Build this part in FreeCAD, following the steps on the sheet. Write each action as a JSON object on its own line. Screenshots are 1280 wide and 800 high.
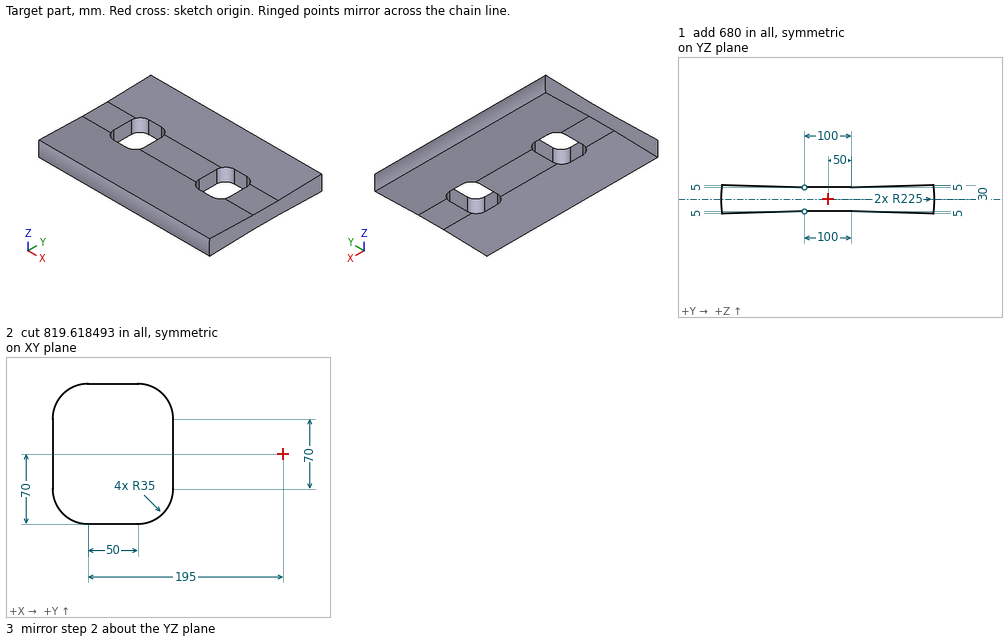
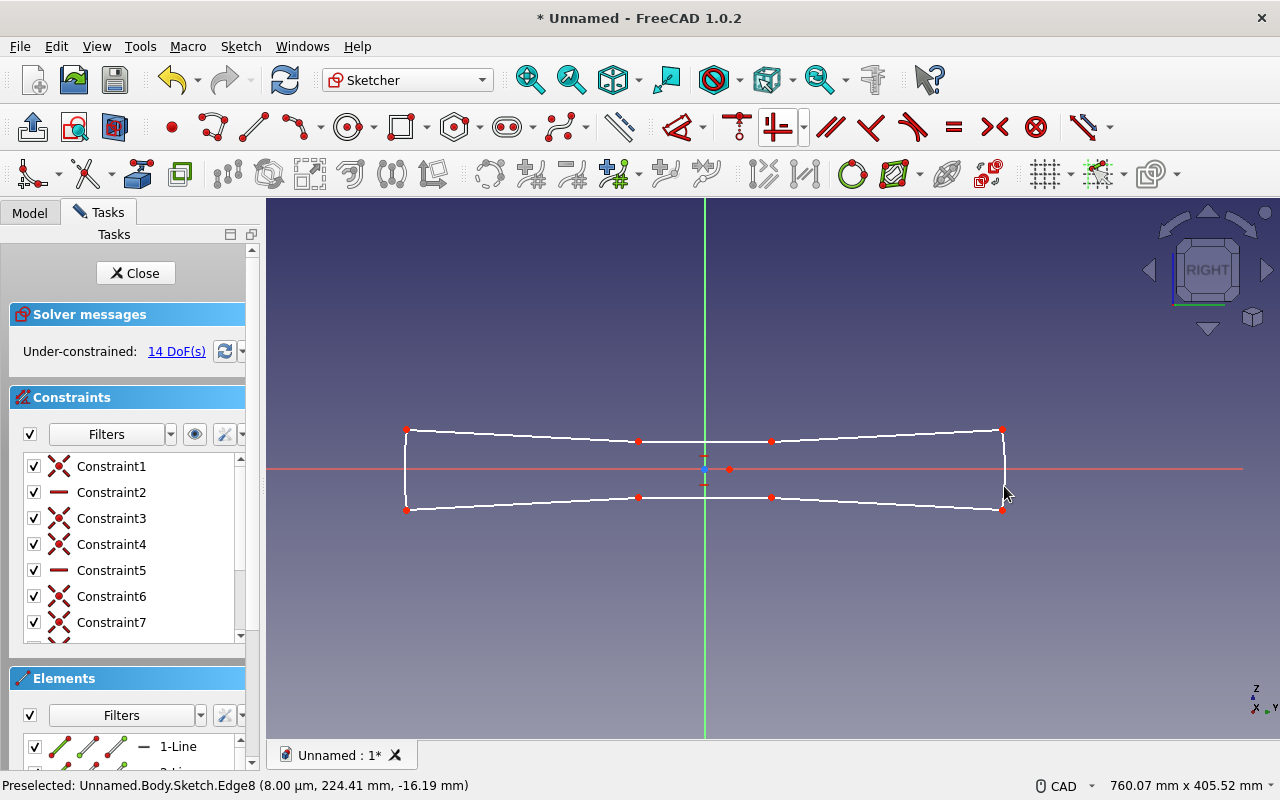
{"action": "left_click_drag", "start_coordinate": [695, 459], "coordinate": [739, 480]}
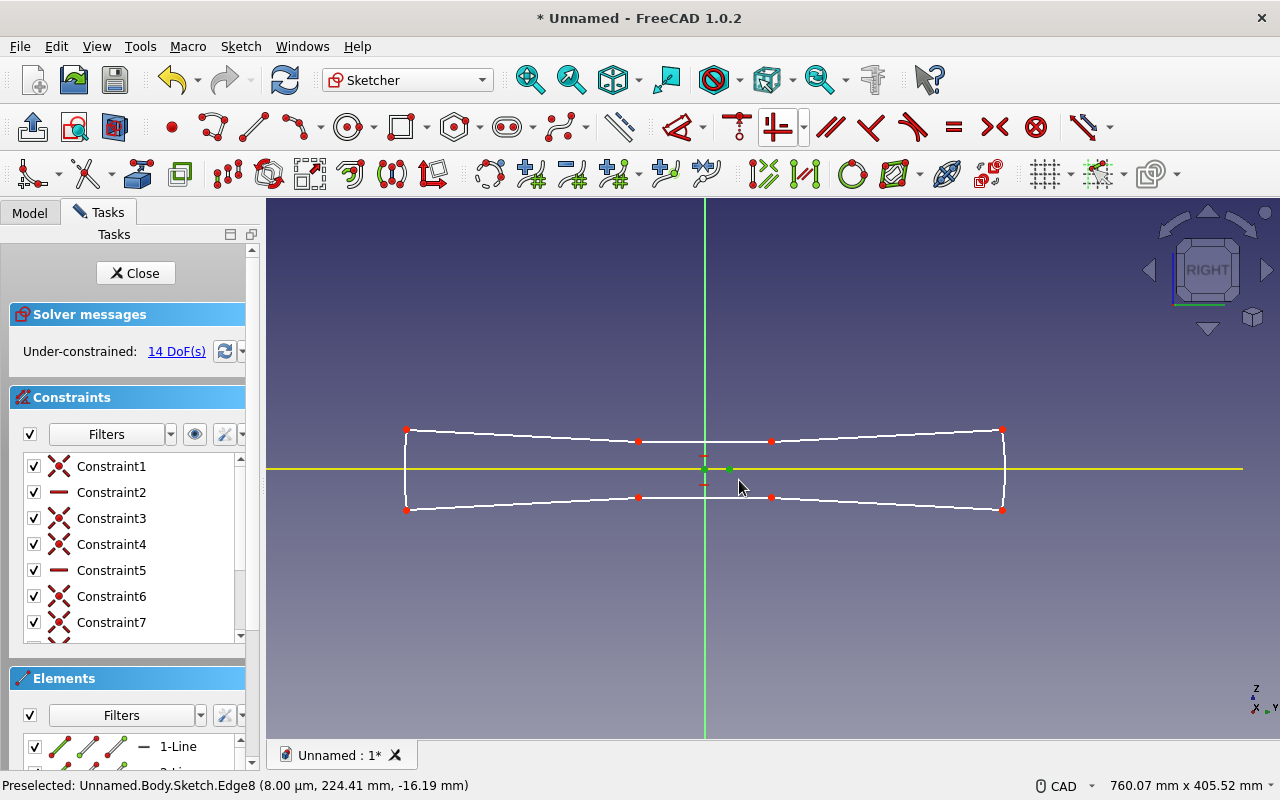
{"action": "left_click", "coordinate": [737, 128]}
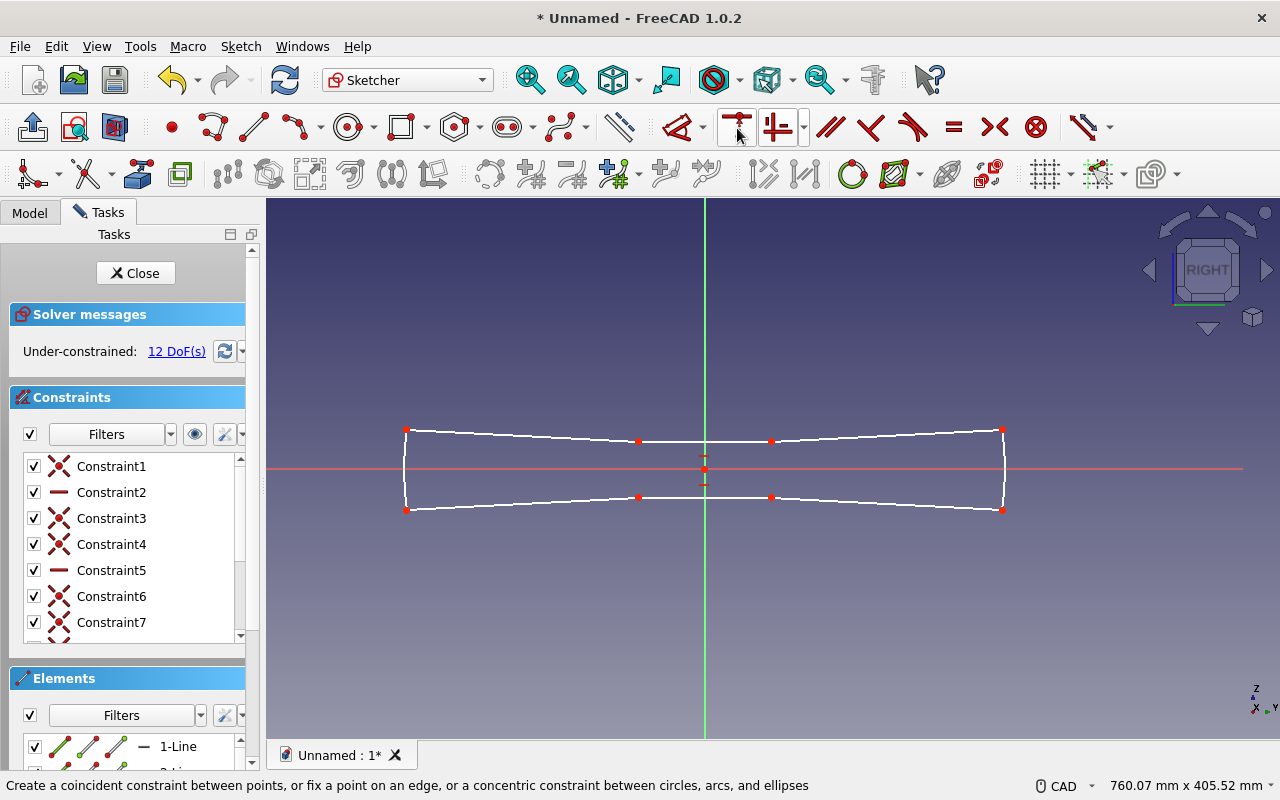
{"action": "left_click", "coordinate": [405, 454]}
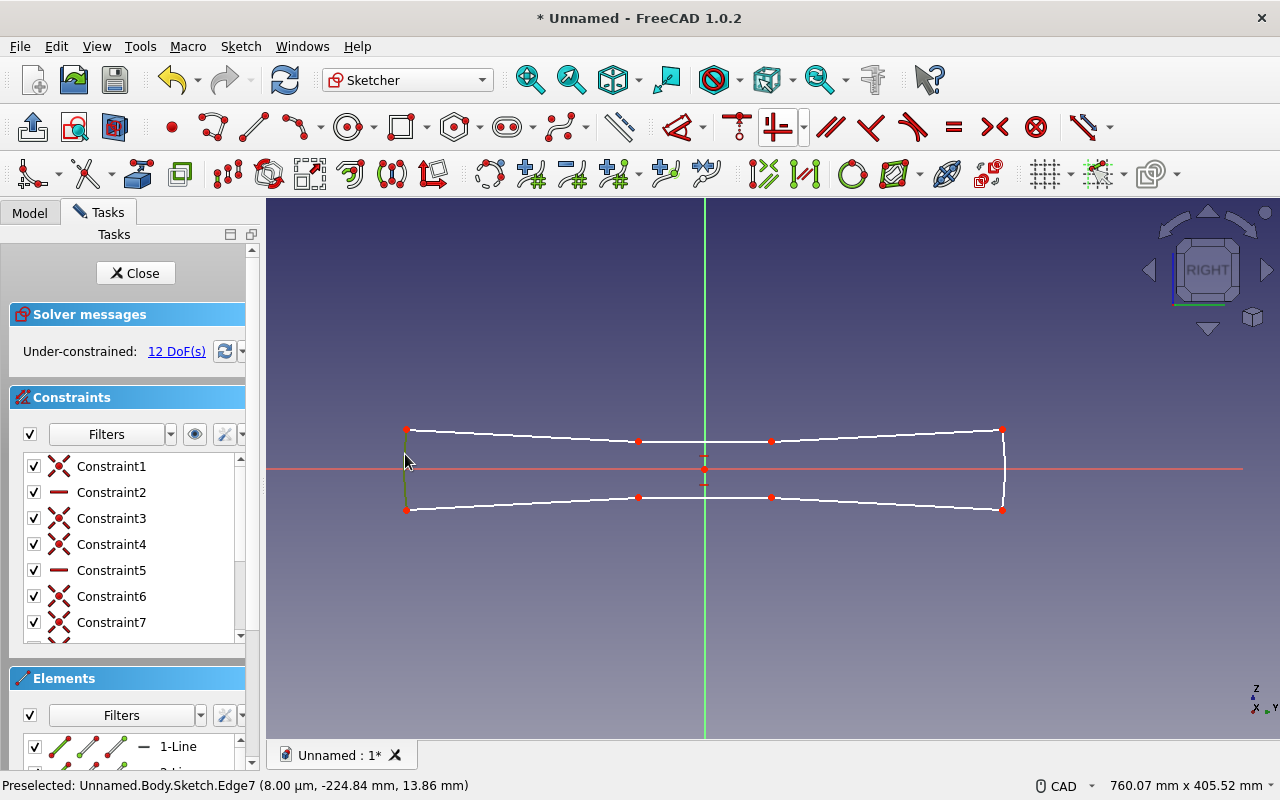
{"action": "left_click", "coordinate": [1004, 486]}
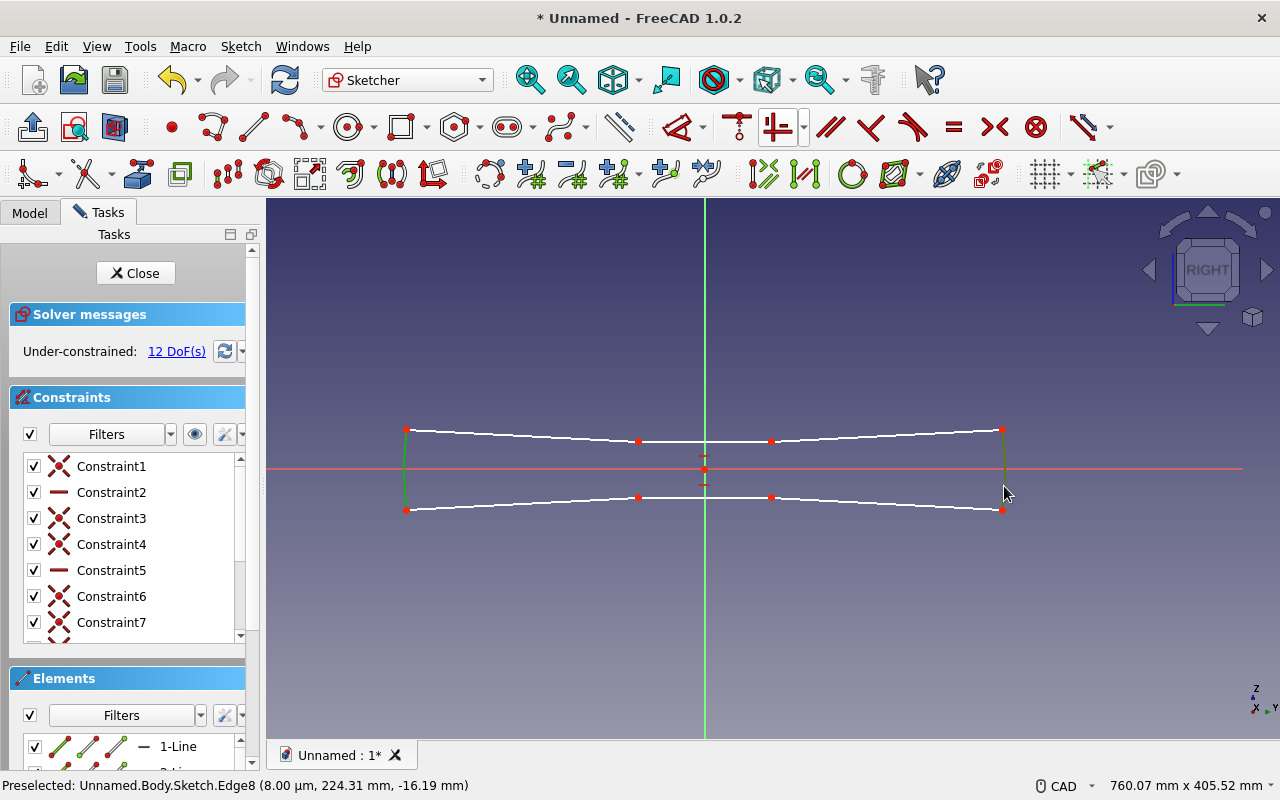
{"action": "left_click", "coordinate": [954, 128]}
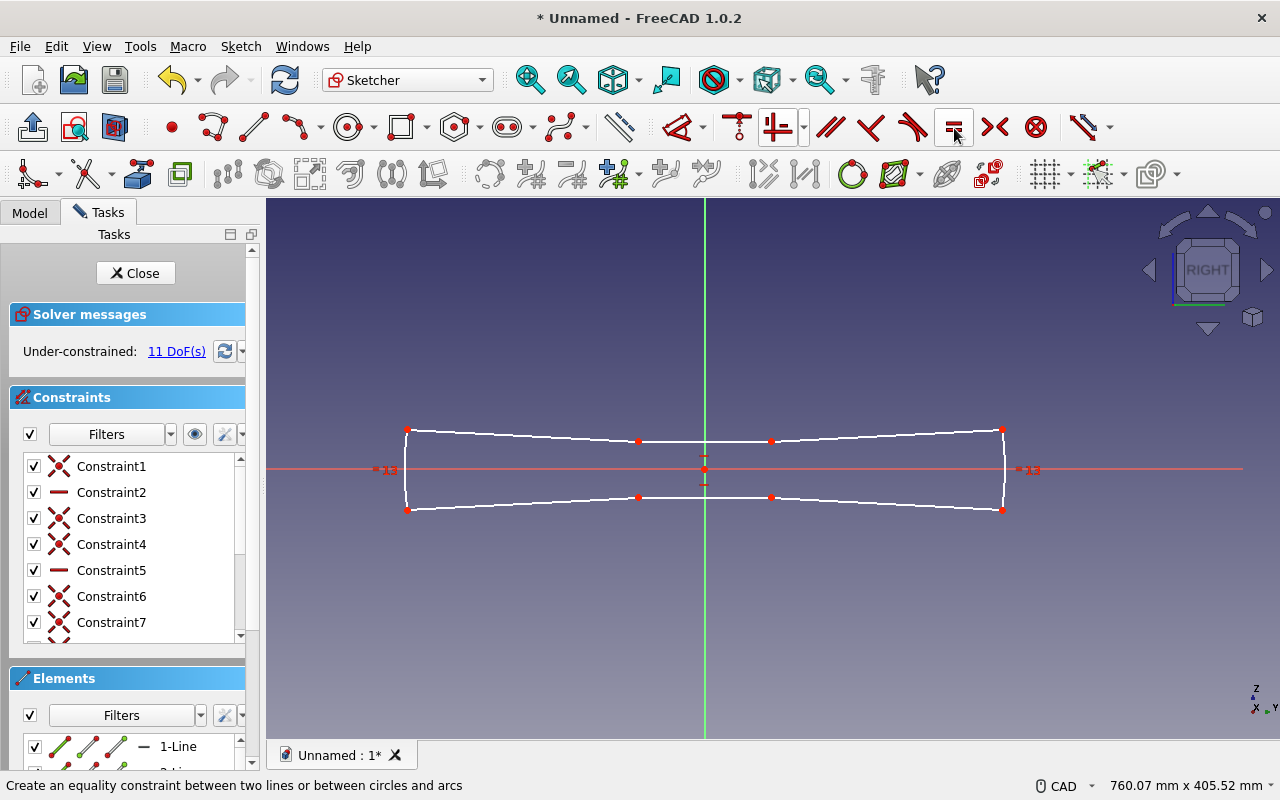
{"action": "left_click", "coordinate": [638, 442]}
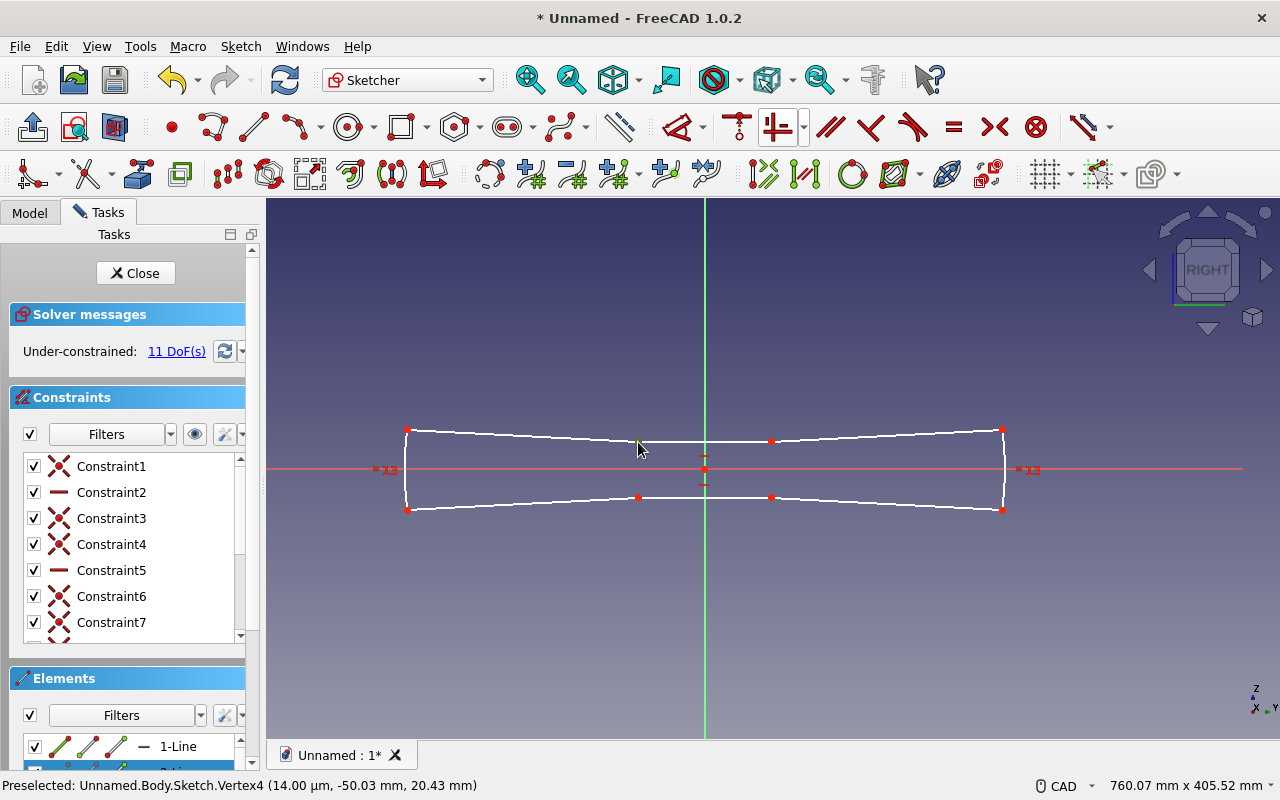
{"action": "left_click", "coordinate": [638, 498]}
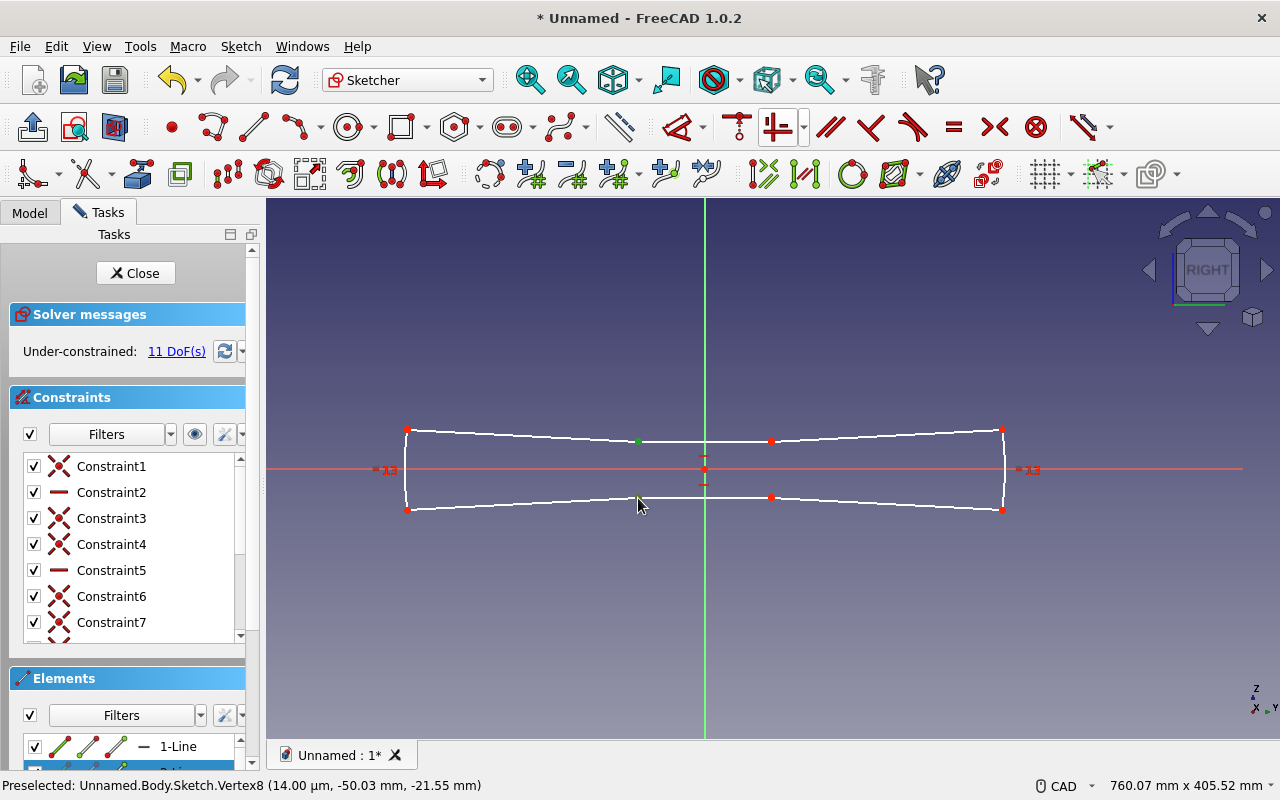
{"action": "left_click", "coordinate": [353, 469]}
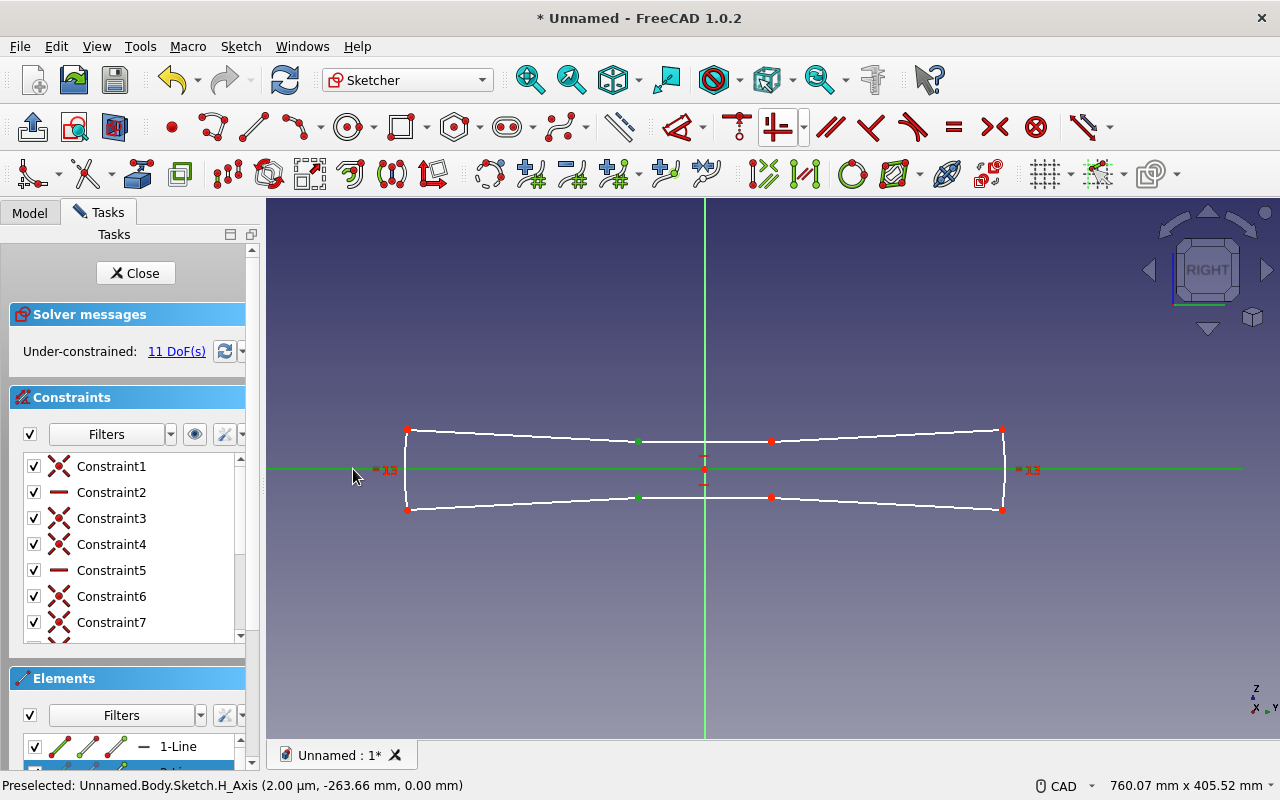
{"action": "key", "text": "s"}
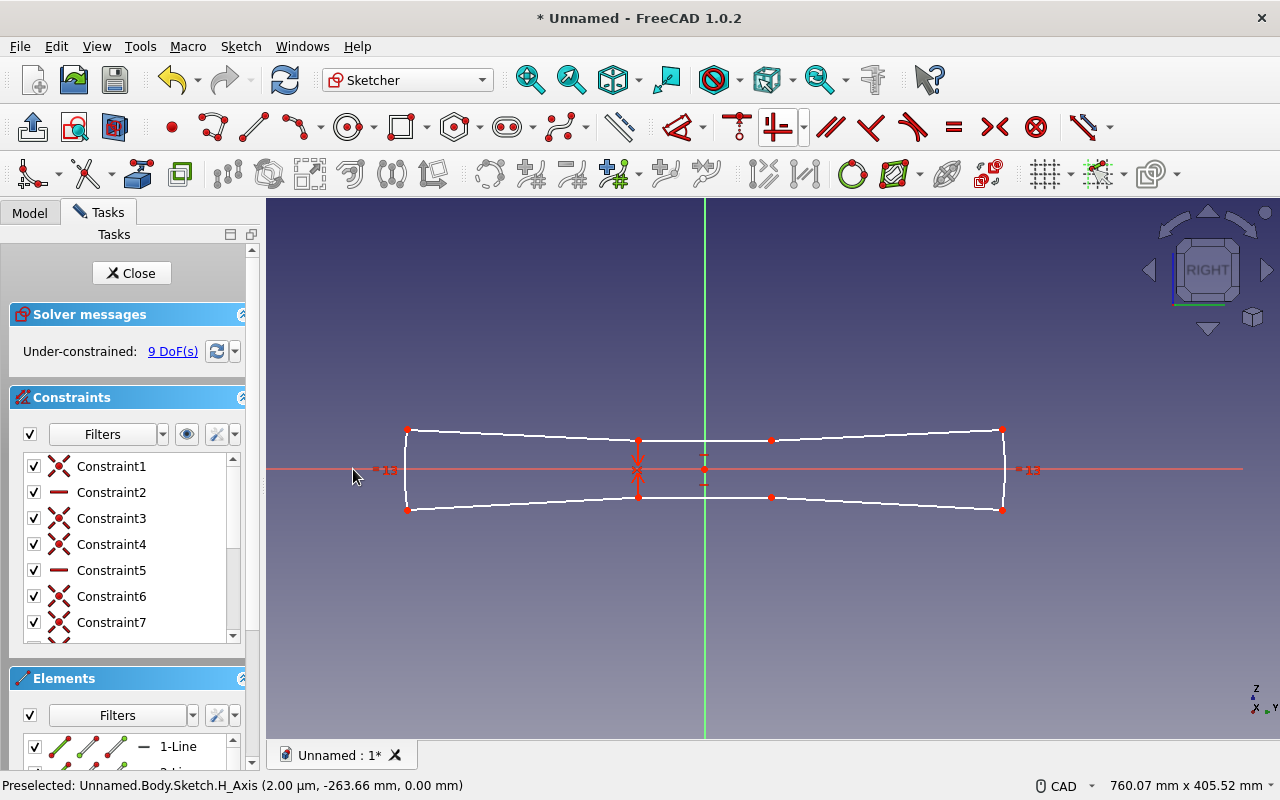
{"action": "key", "text": "d"}